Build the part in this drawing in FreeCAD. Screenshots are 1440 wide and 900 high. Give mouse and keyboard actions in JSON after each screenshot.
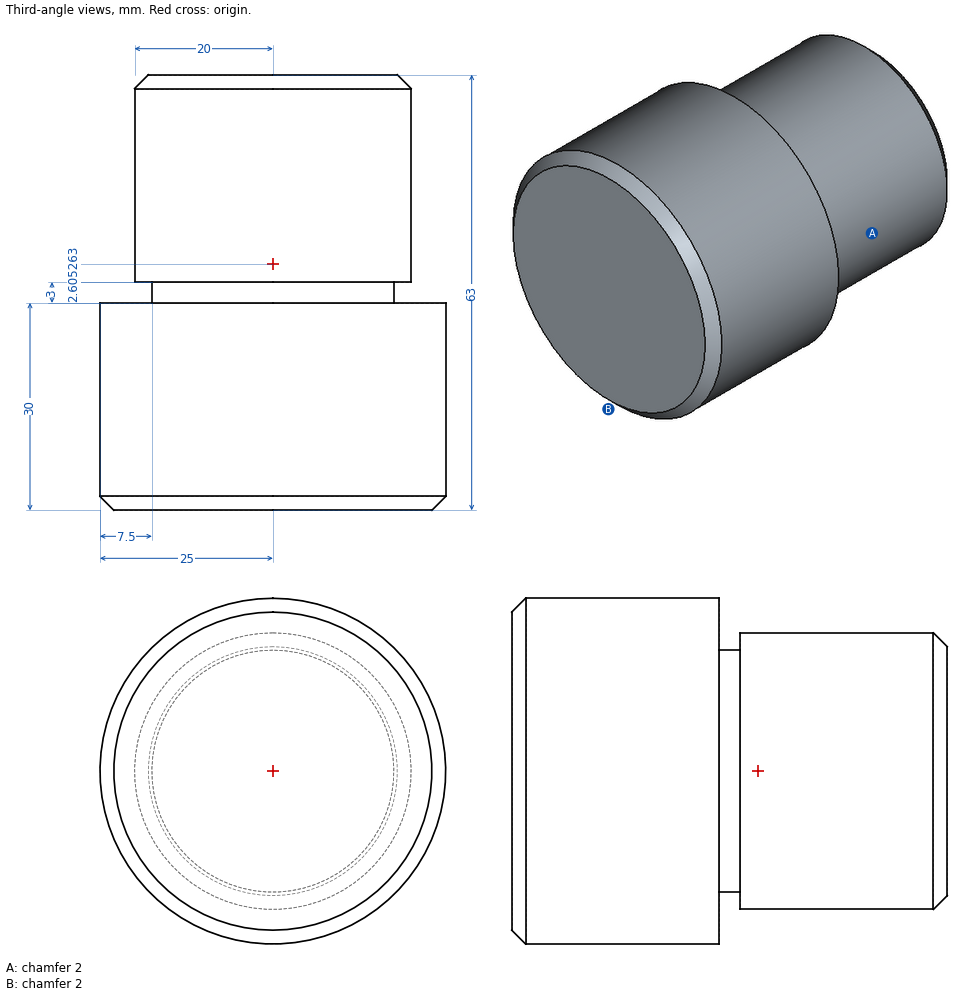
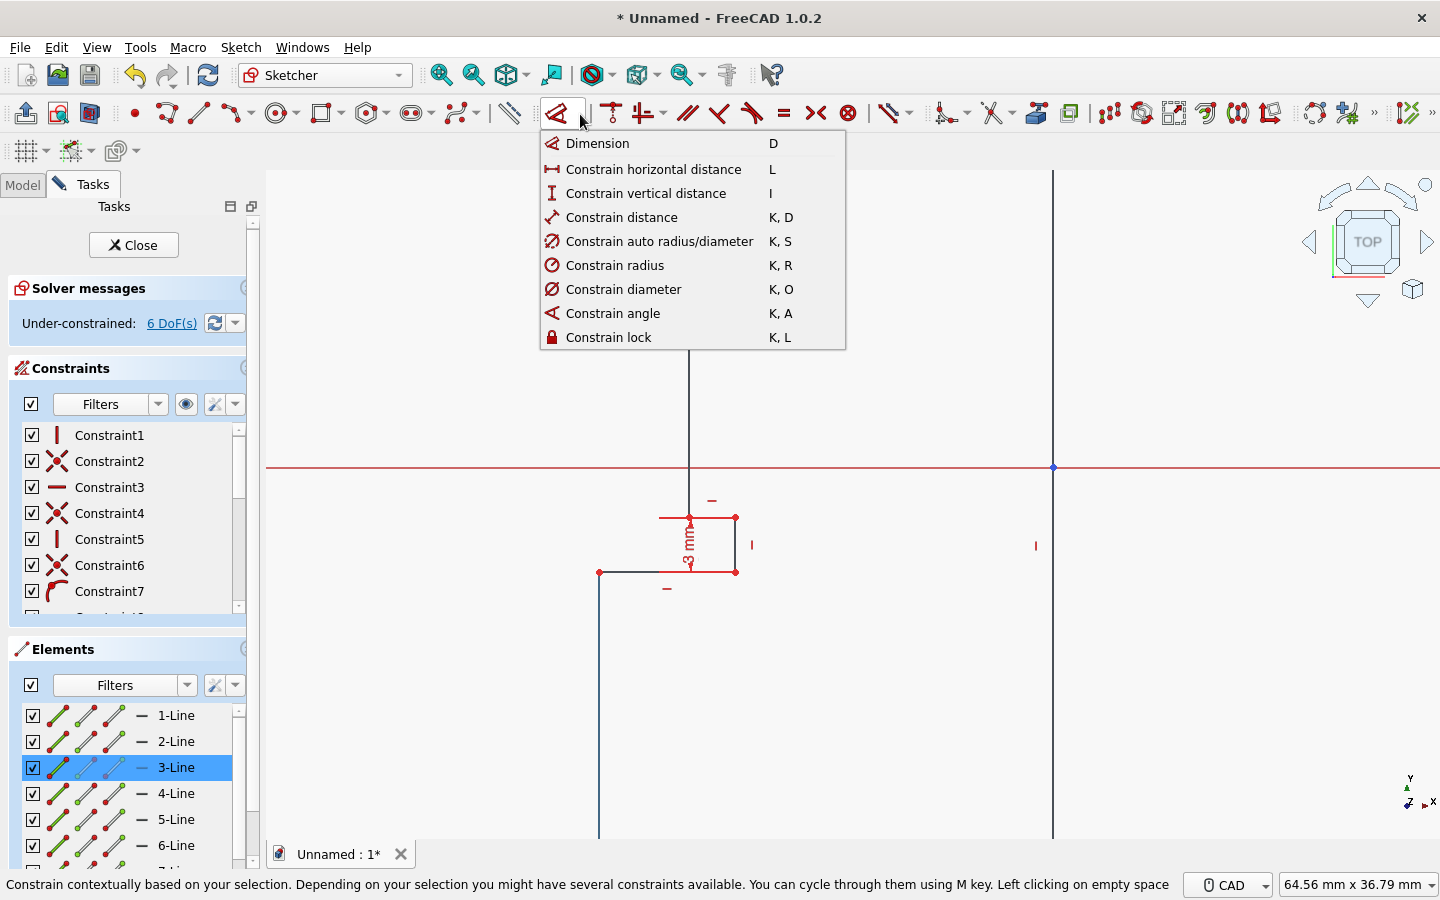
{"action": "left_click", "coordinate": [693, 193]}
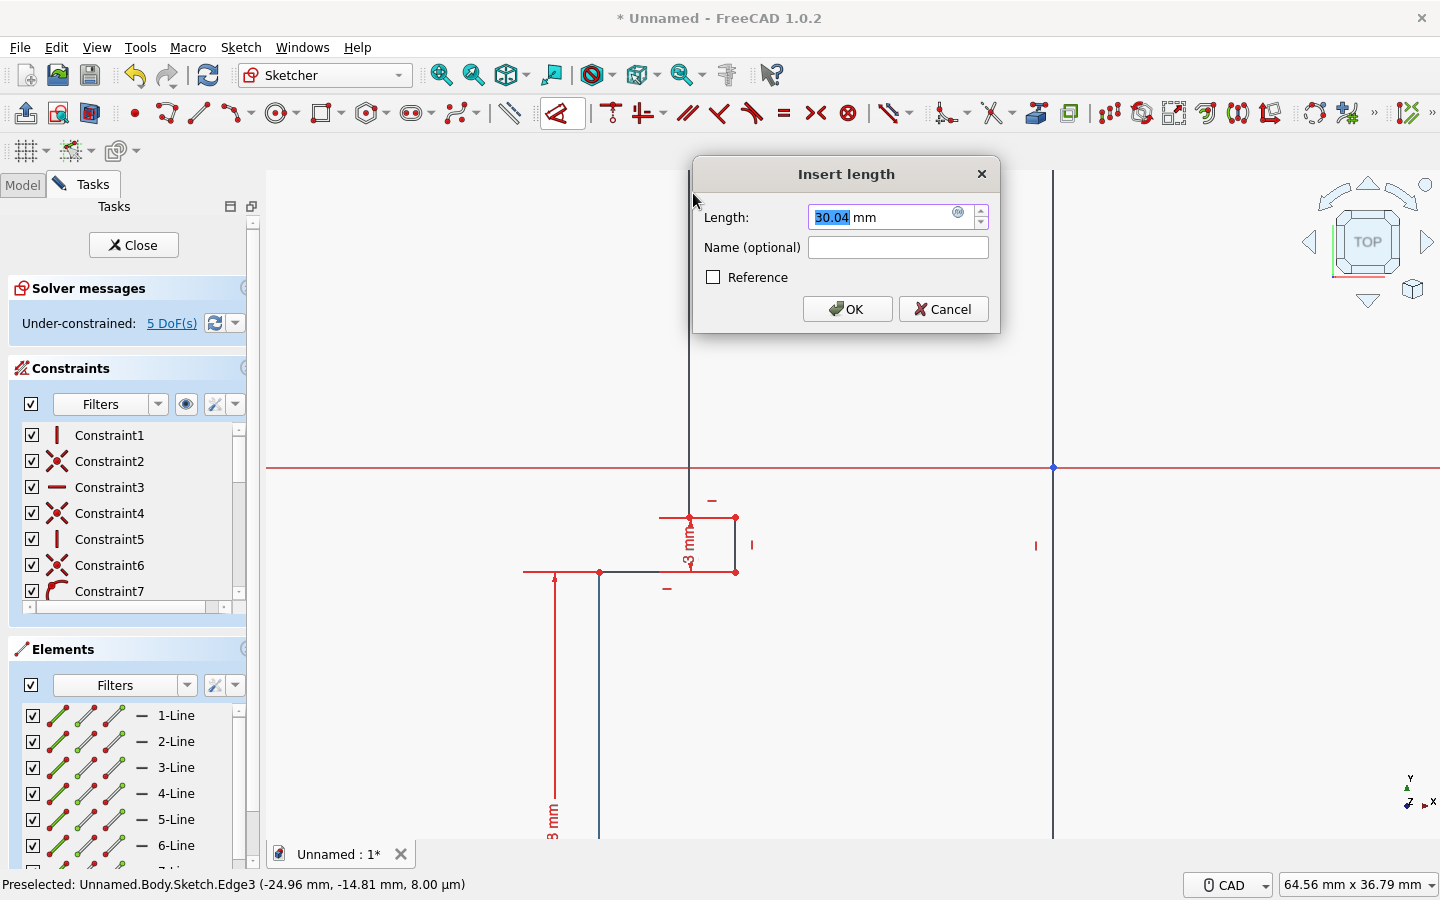
{"action": "type", "text": "30"}
{"action": "key", "text": "Return"}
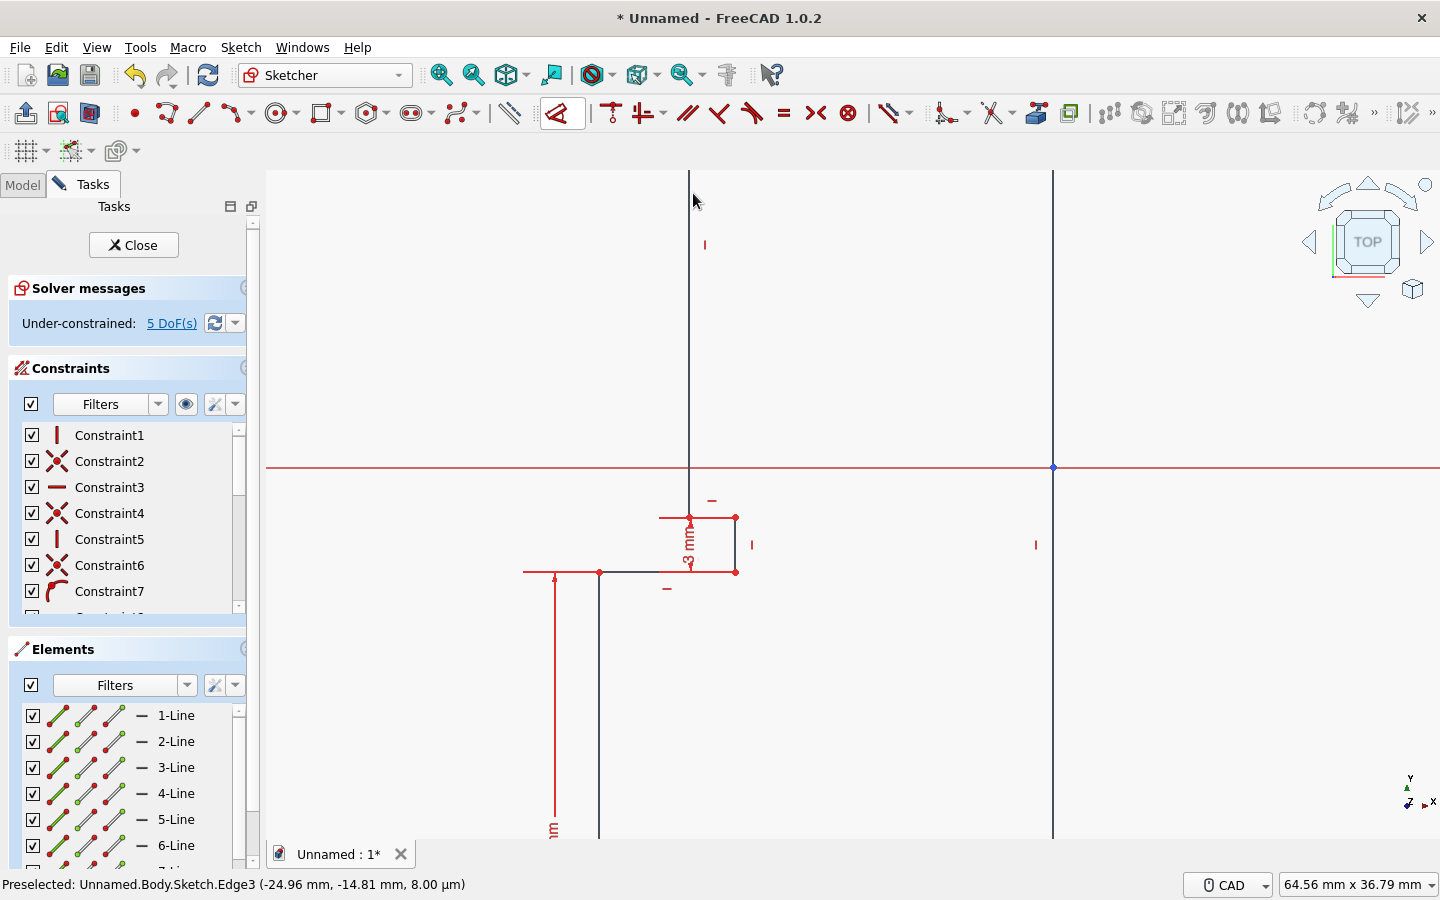
{"action": "scroll", "coordinate": [760, 483], "scroll_direction": "down", "scroll_amount": 5}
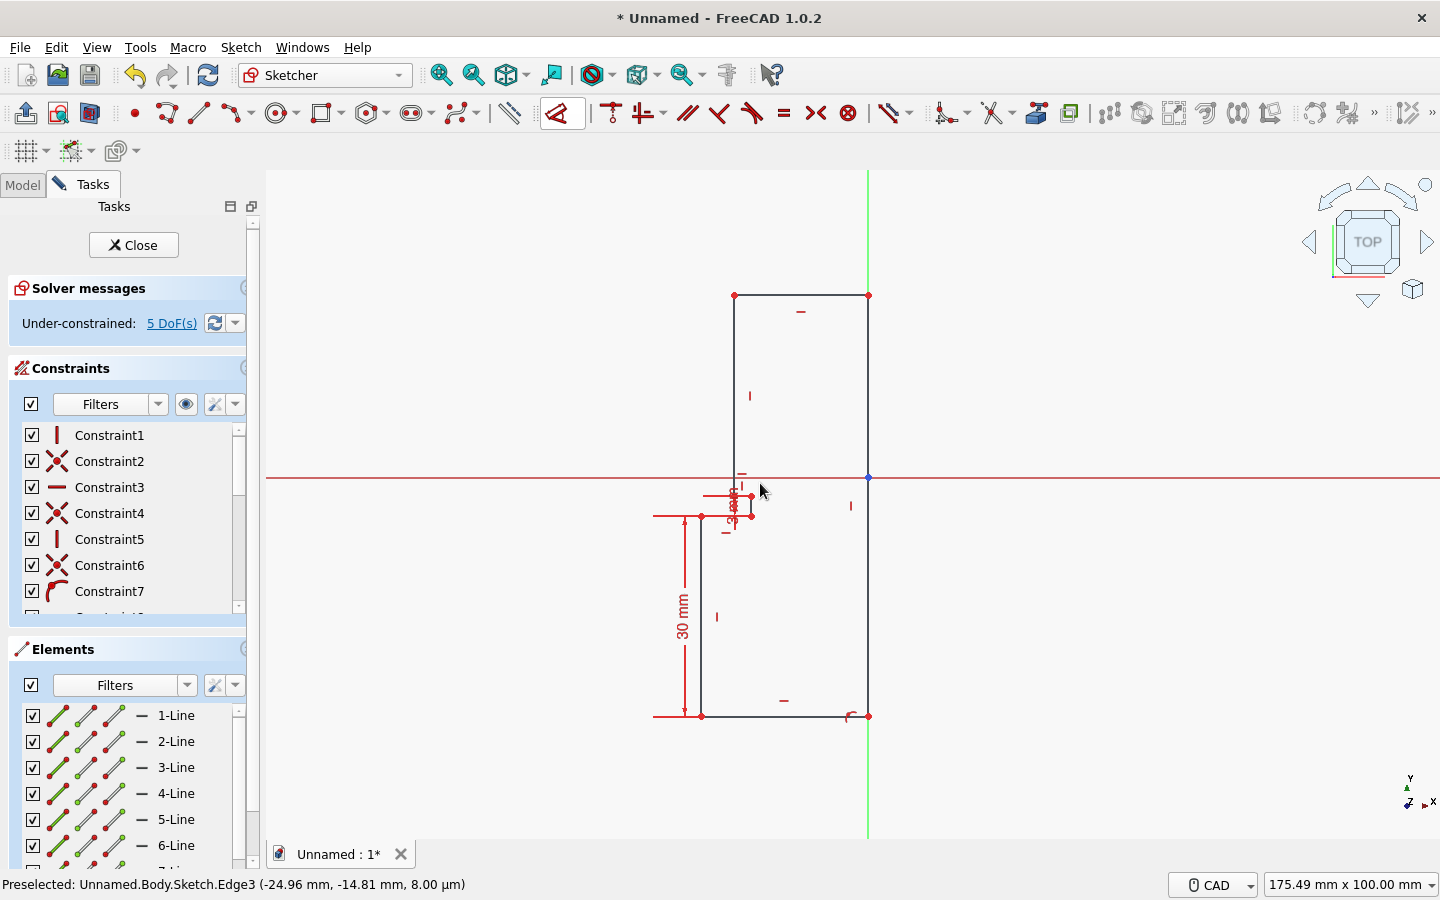
{"action": "left_click", "coordinate": [751, 717]}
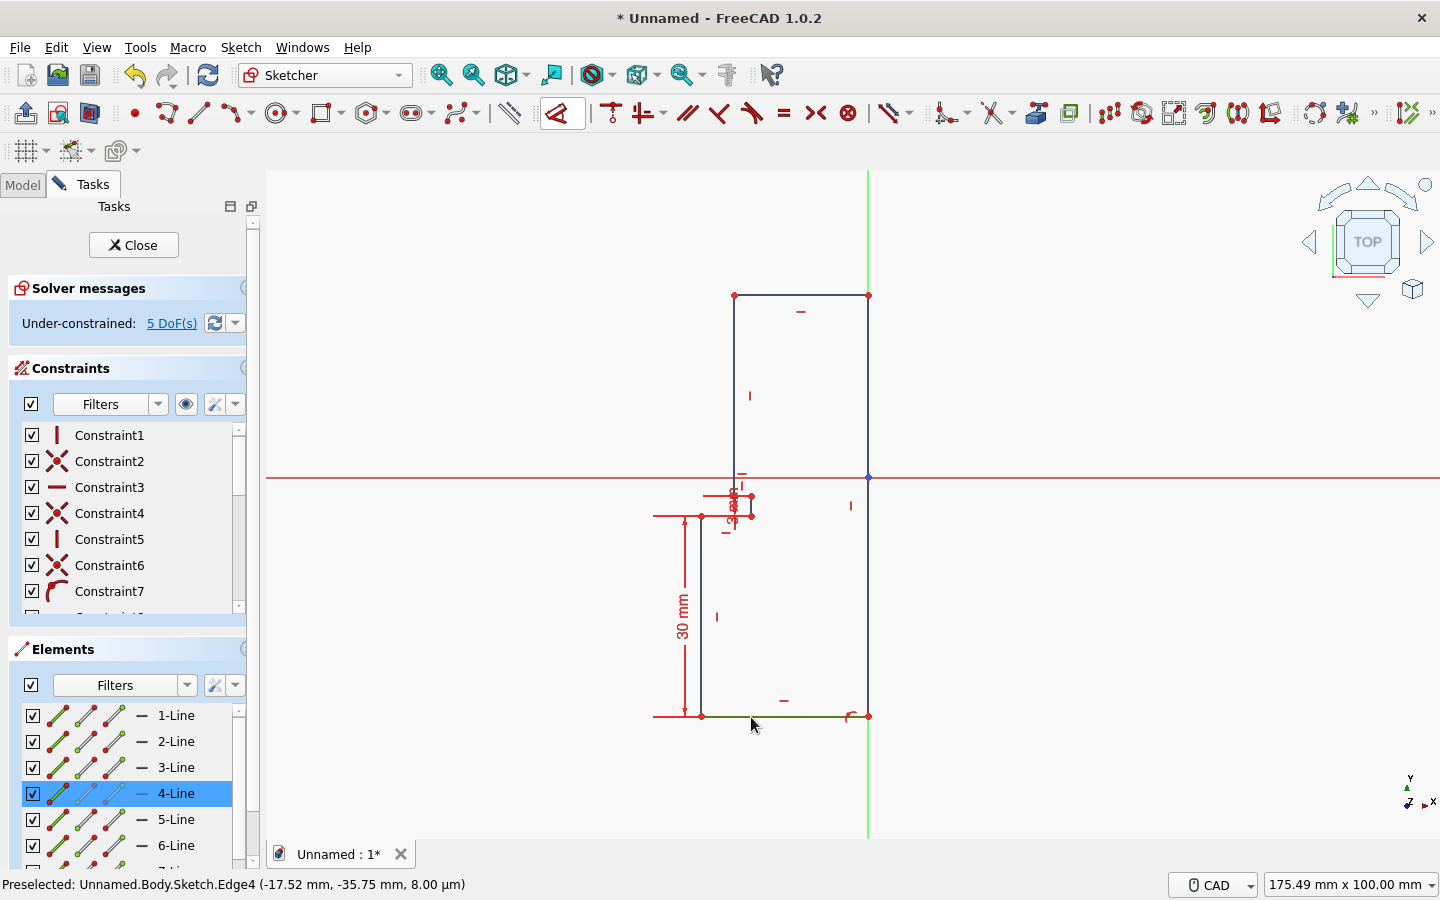
{"action": "key", "text": "l"}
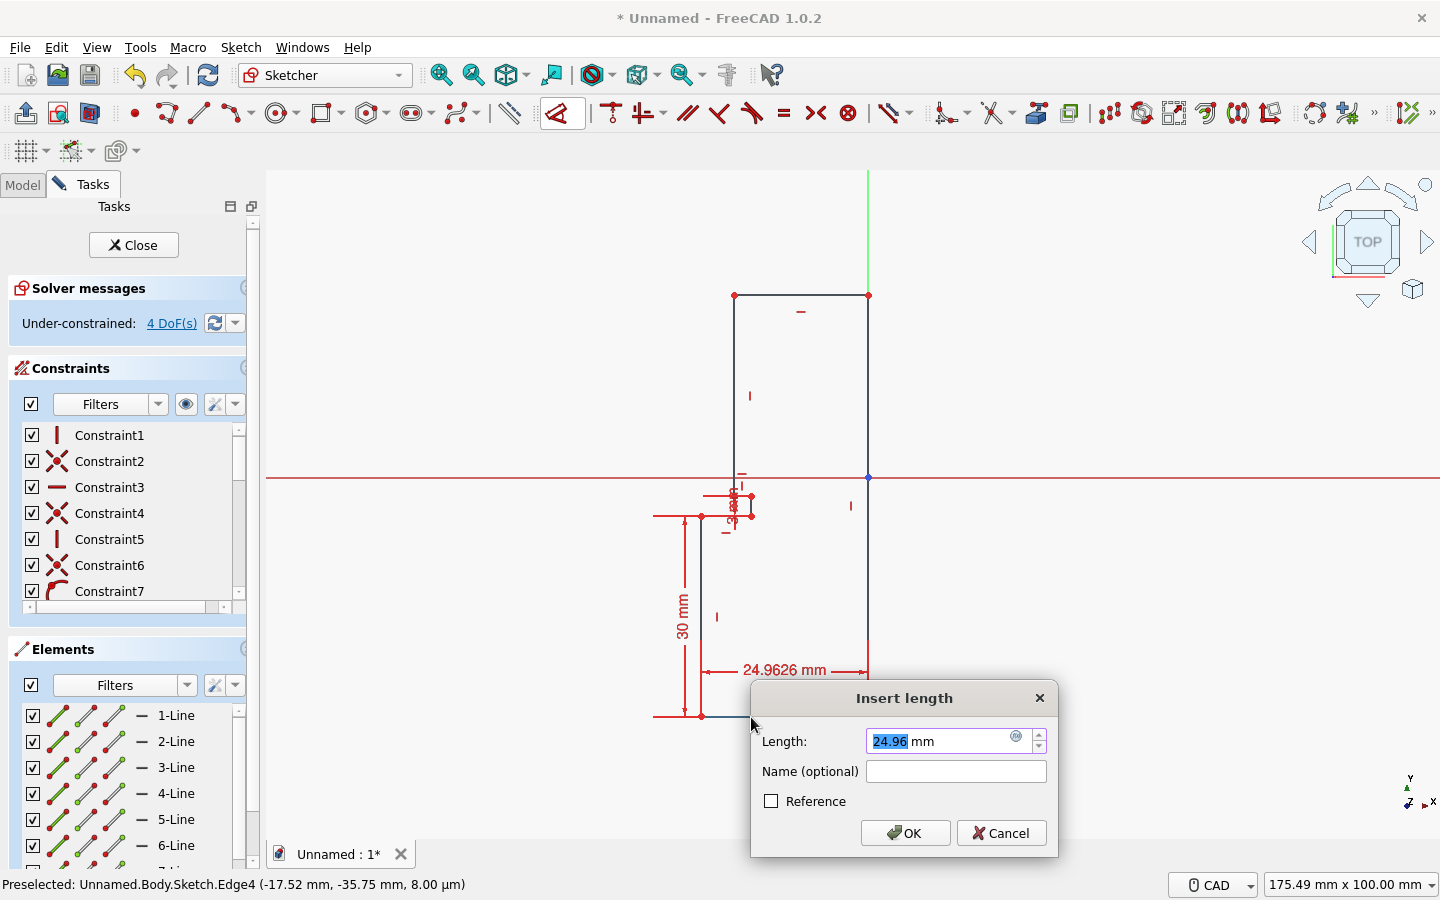
{"action": "type", "text": "25"}
{"action": "key", "text": "Return"}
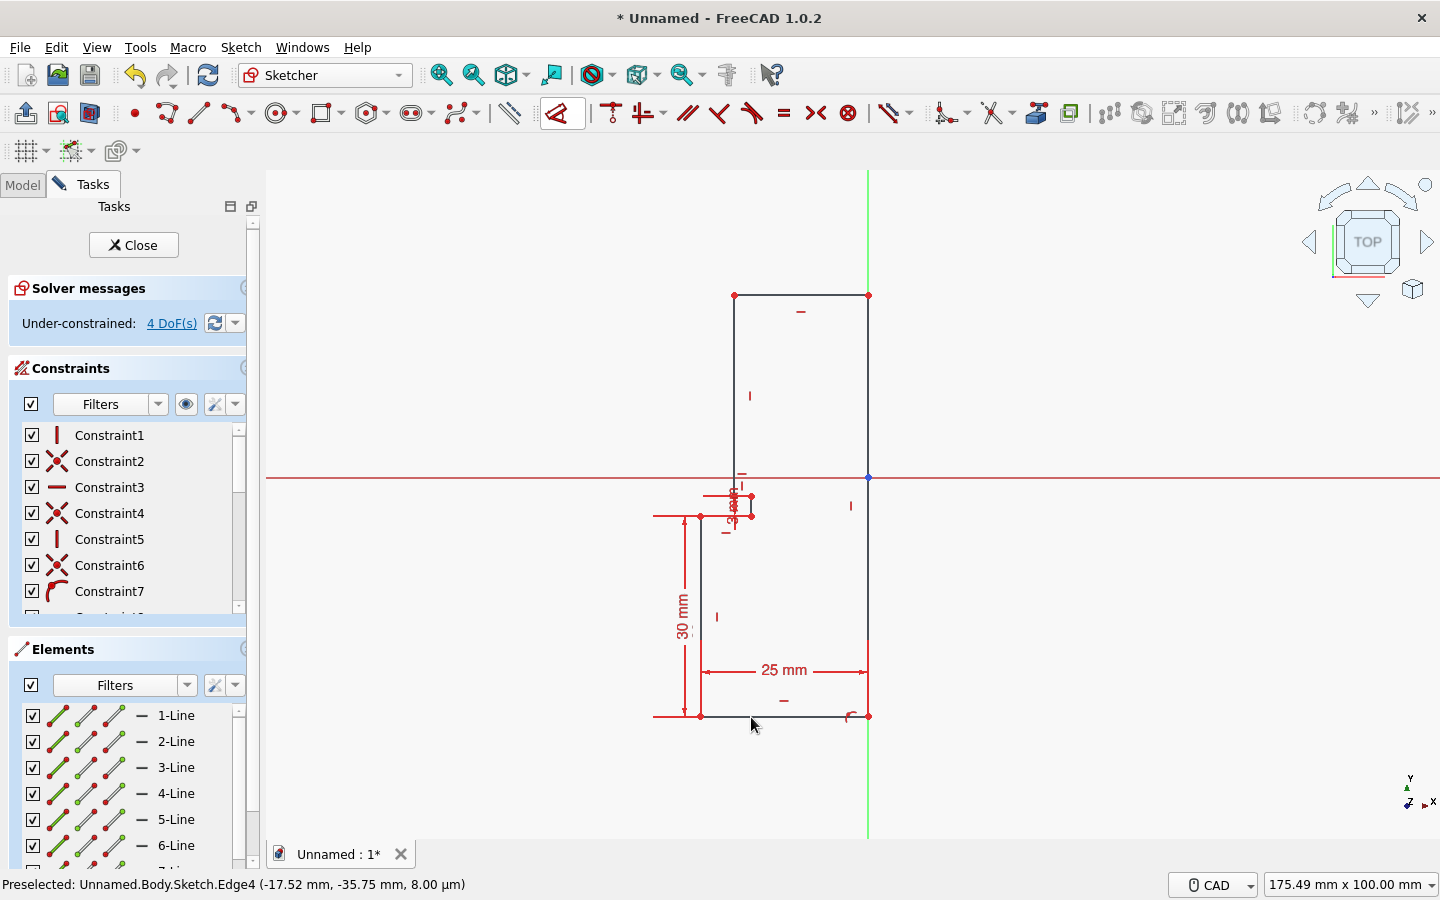
{"action": "left_click", "coordinate": [868, 590]}